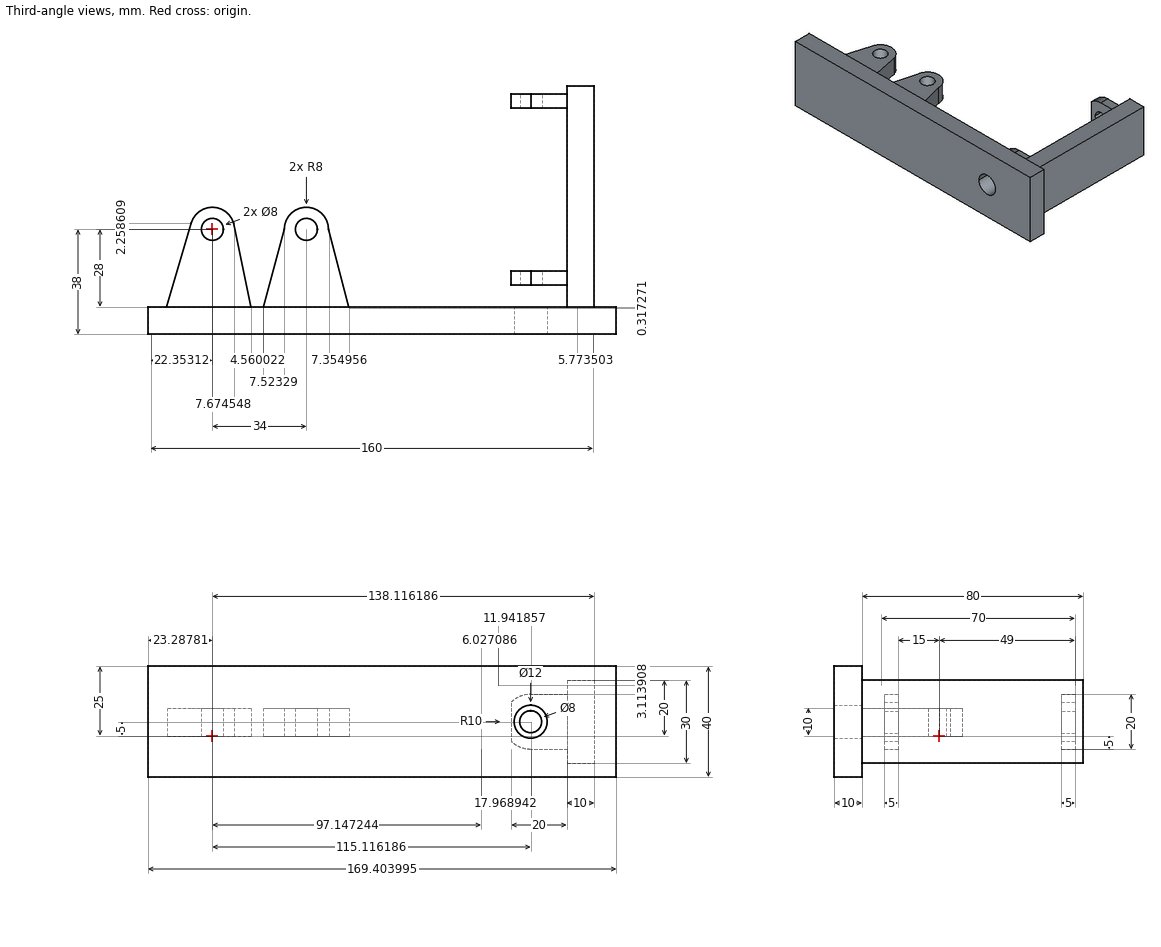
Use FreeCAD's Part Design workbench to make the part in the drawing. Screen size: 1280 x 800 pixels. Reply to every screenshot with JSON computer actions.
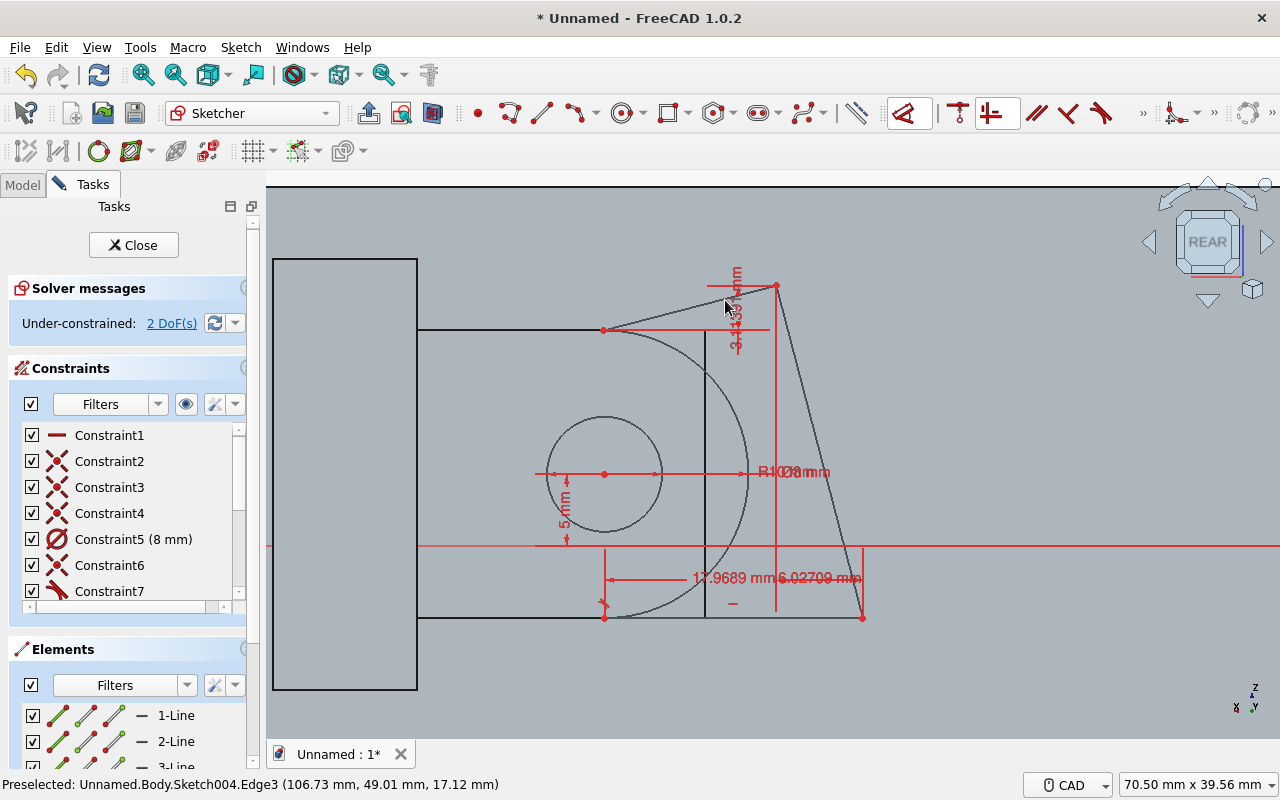
{"action": "left_click", "coordinate": [863, 618]}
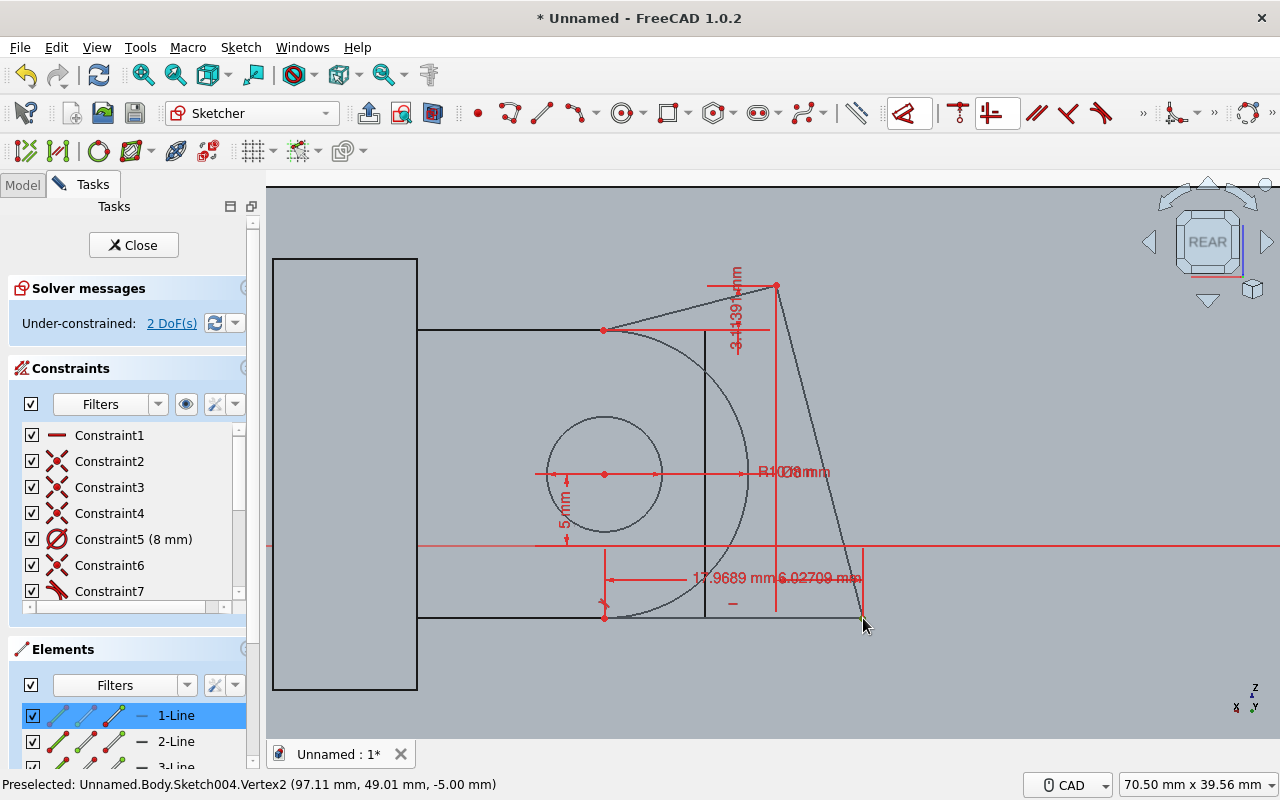
{"action": "left_click", "coordinate": [926, 114]}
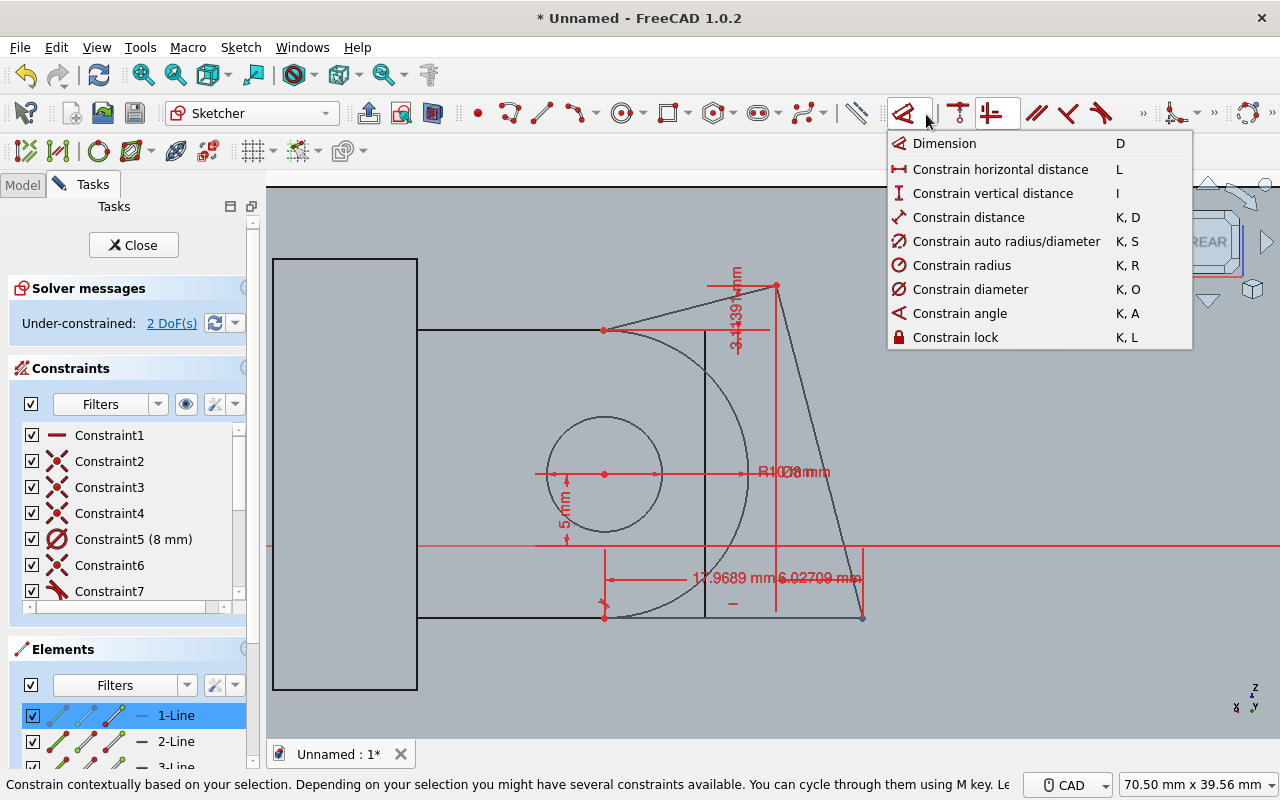
{"action": "left_click", "coordinate": [1040, 169]}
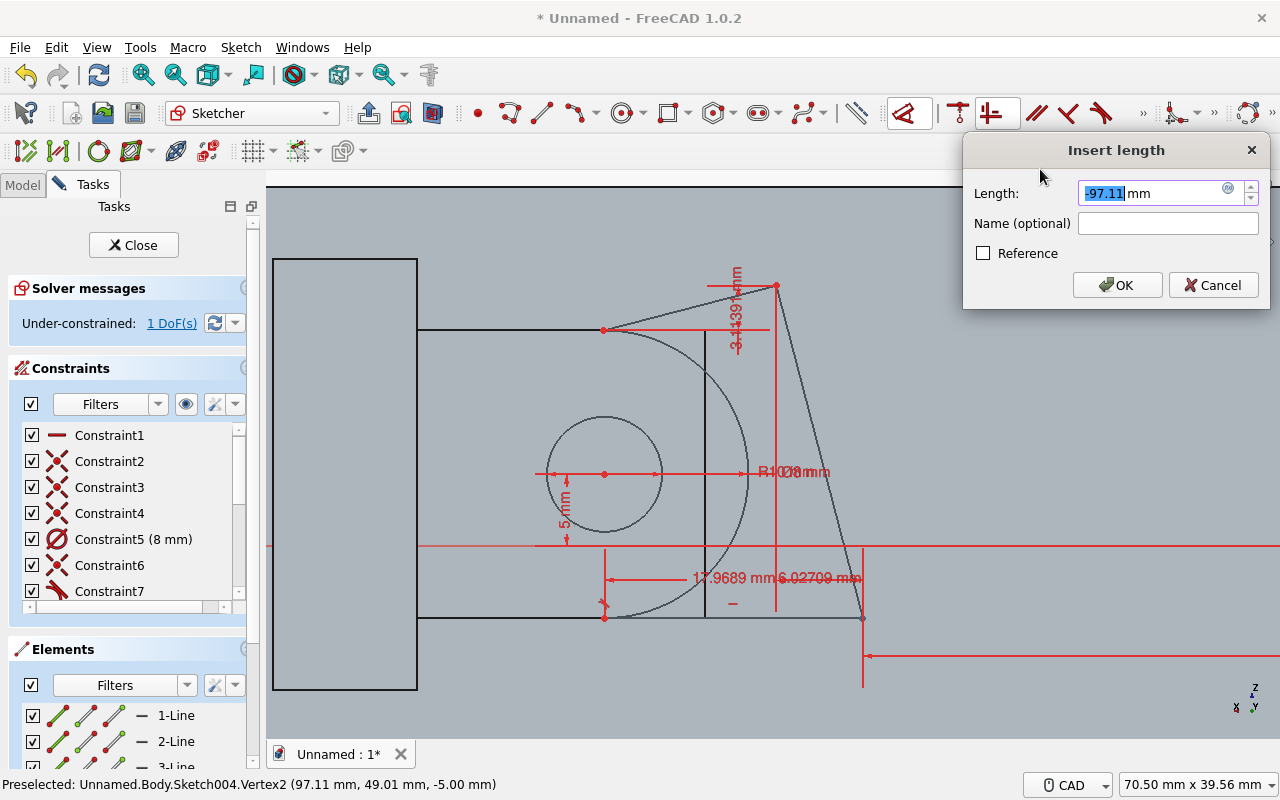
{"action": "type", "text": "-97.147244"}
{"action": "key", "text": "Return"}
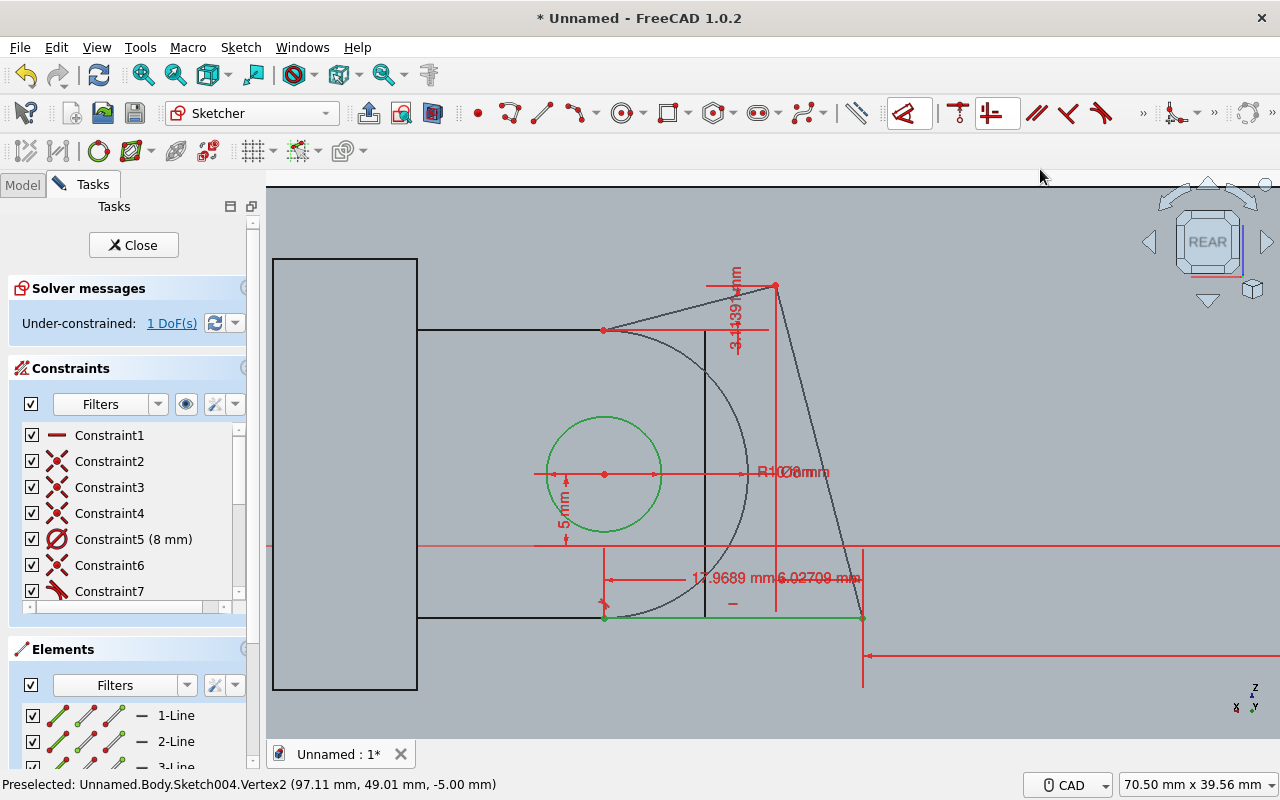
{"action": "left_click", "coordinate": [724, 299]}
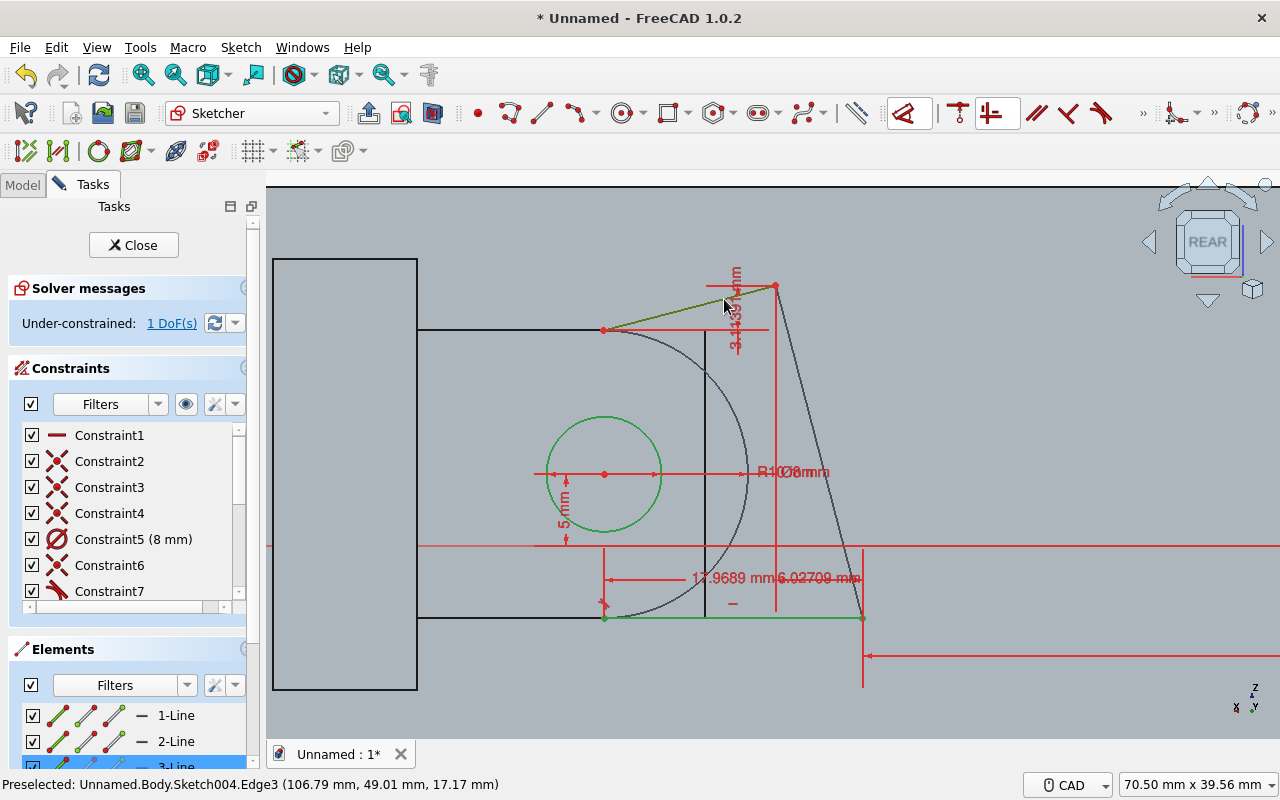
{"action": "key", "text": "l"}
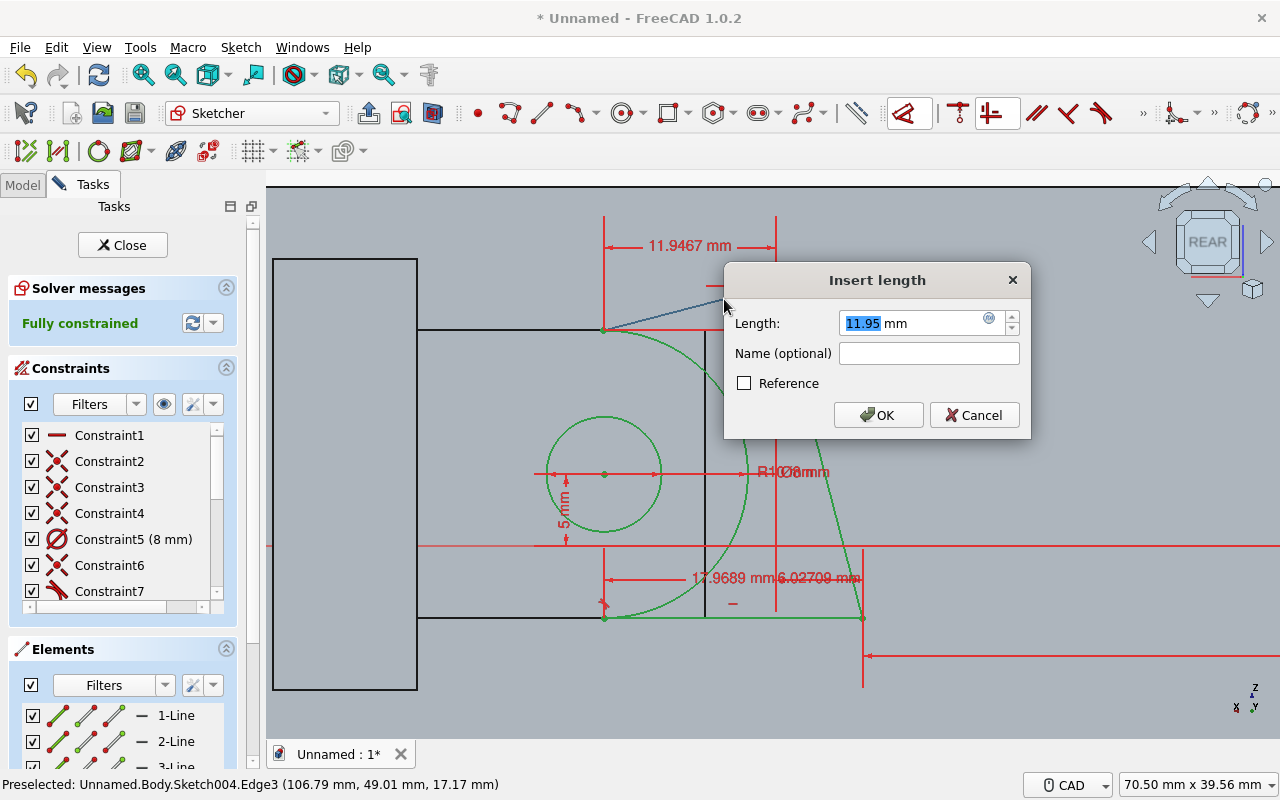
{"action": "type", "text": "11.941857"}
{"action": "key", "text": "Return"}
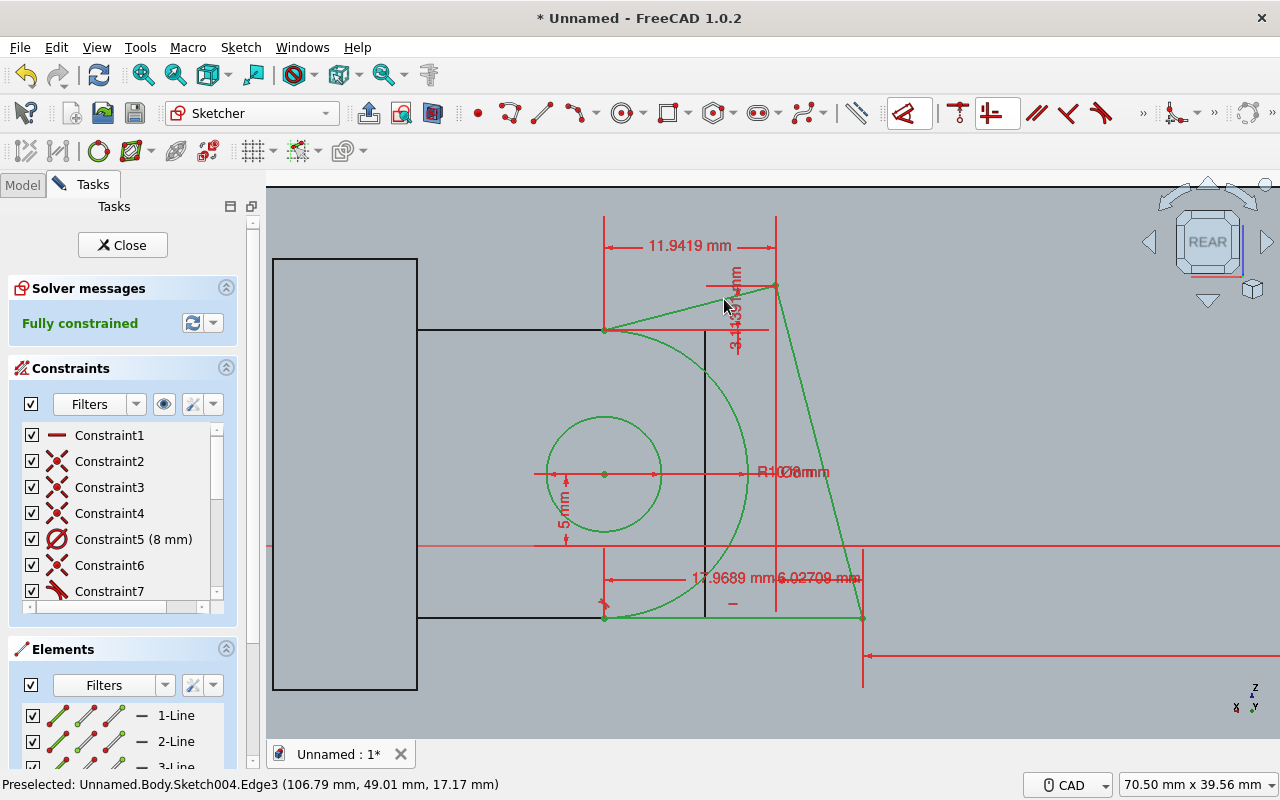
{"action": "left_click", "coordinate": [123, 245]}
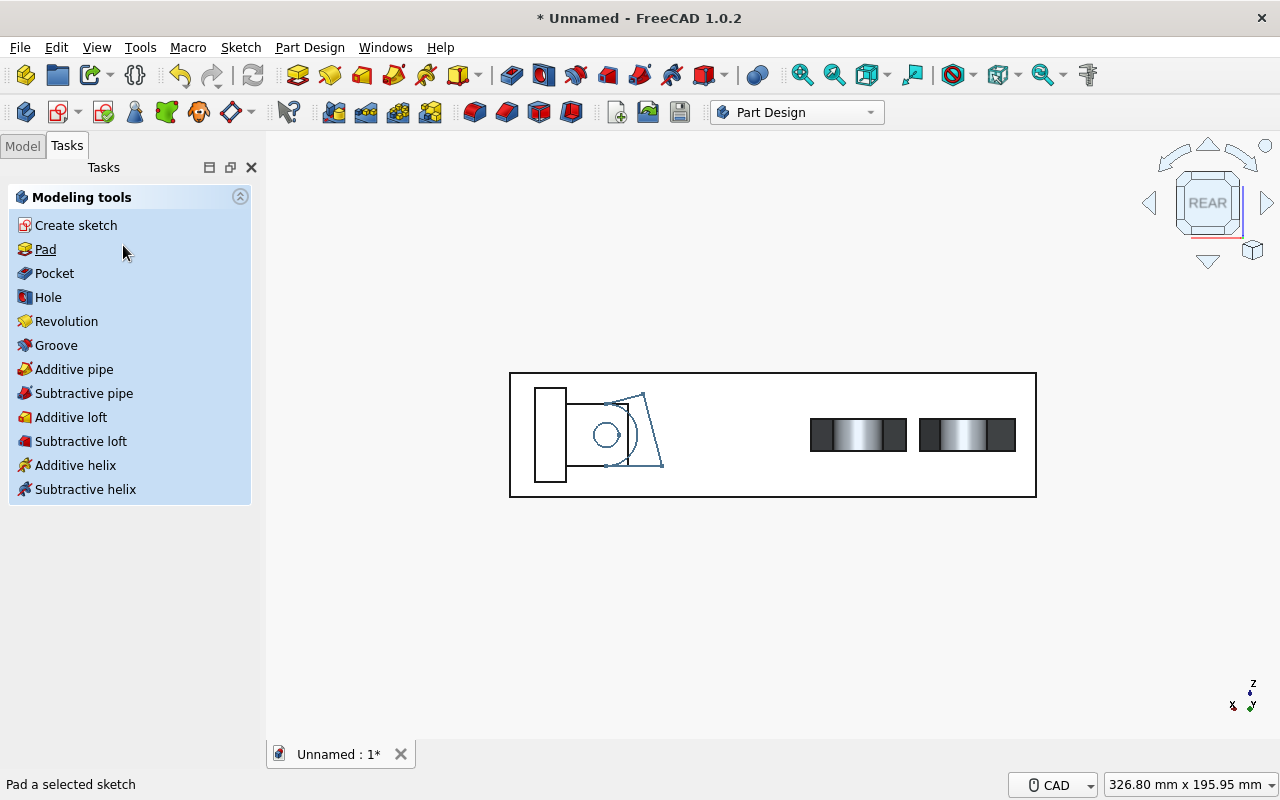
{"action": "left_click", "coordinate": [512, 76]}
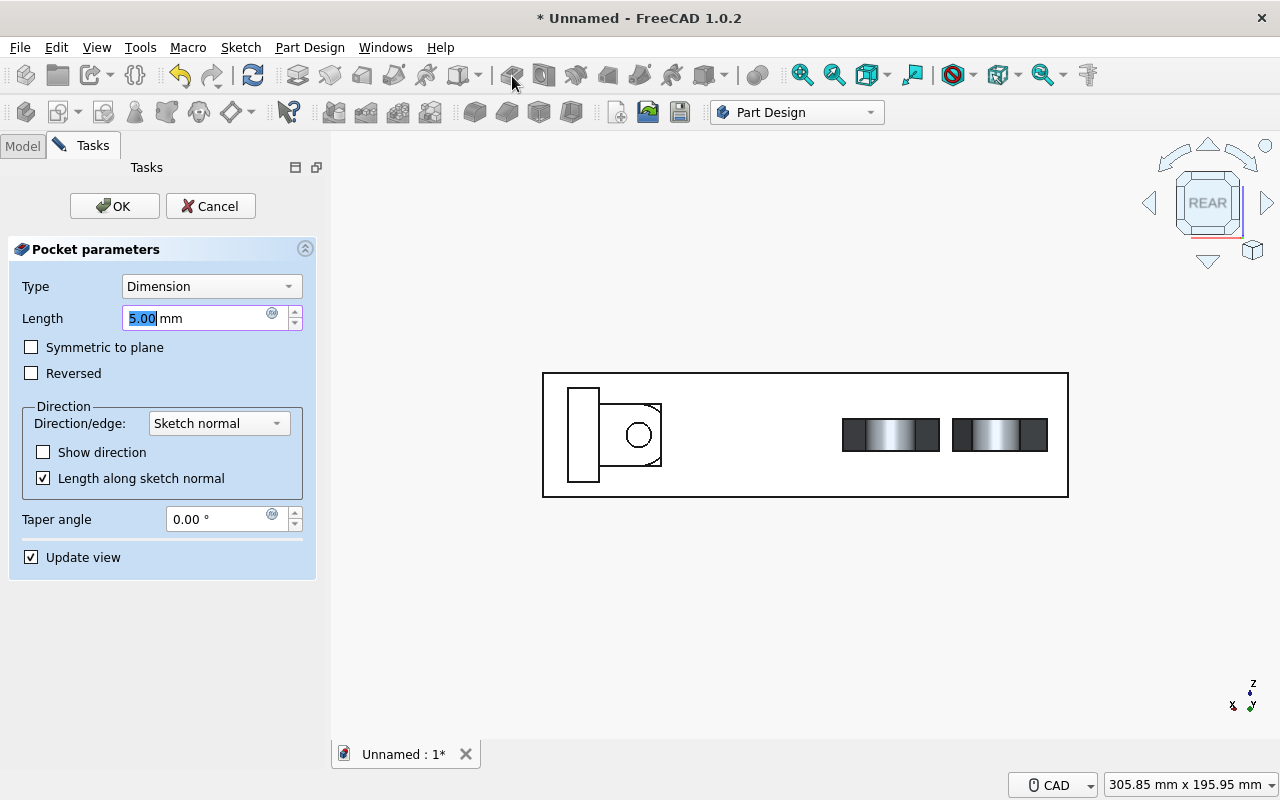
{"action": "type", "text": "70"}
{"action": "key", "text": "Tab"}